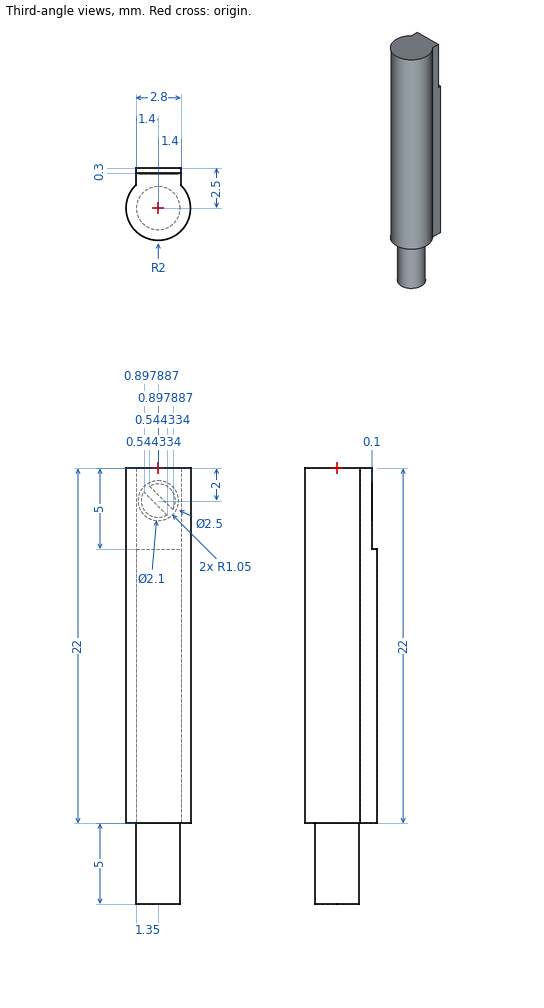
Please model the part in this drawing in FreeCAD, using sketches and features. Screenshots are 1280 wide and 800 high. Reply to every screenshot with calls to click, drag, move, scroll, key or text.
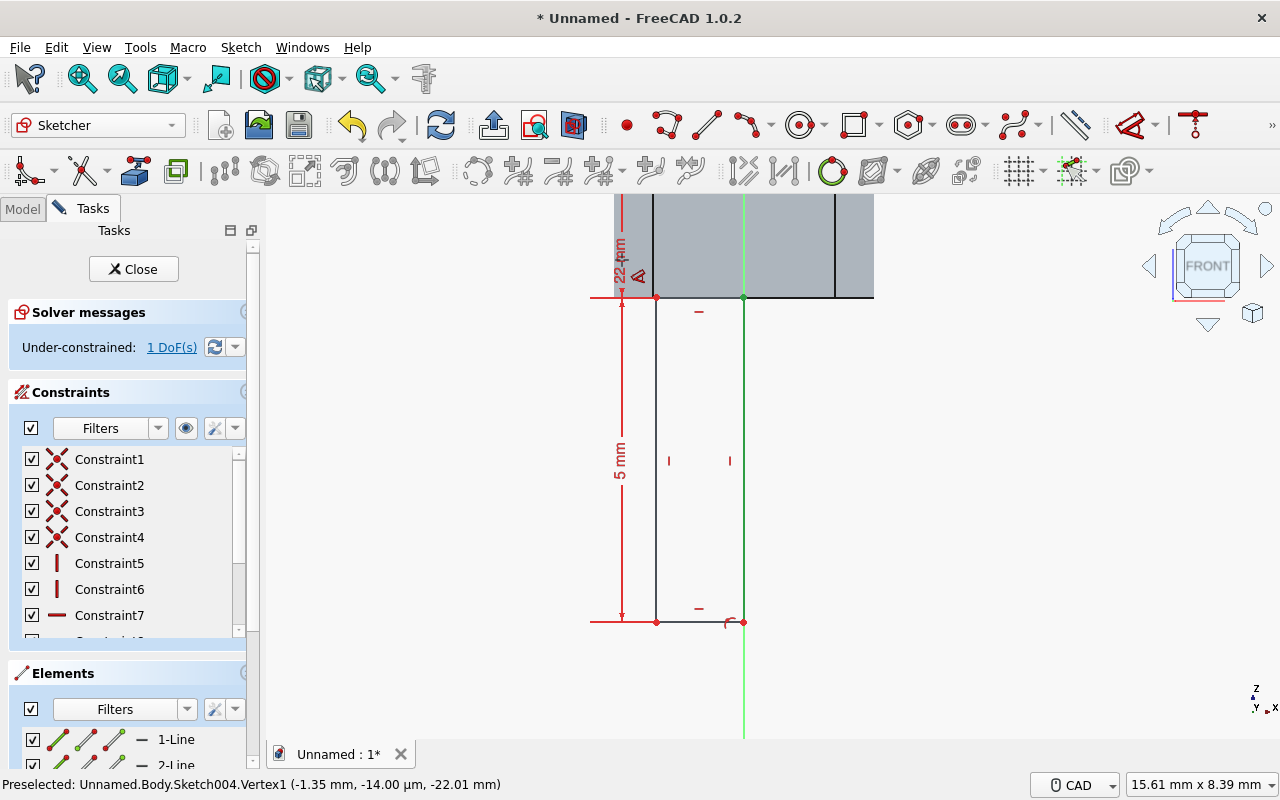
click(682, 622)
click(700, 656)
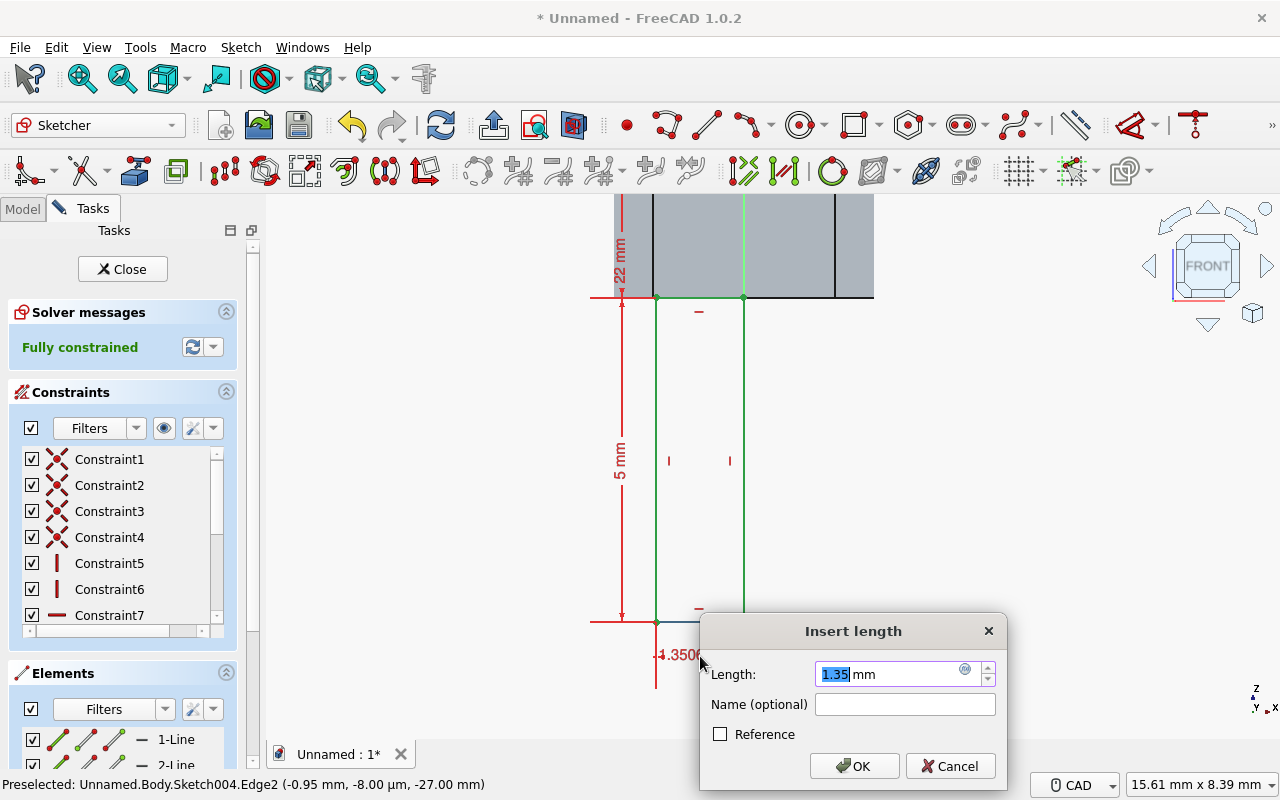
text(1.35)
key(Return)
key(Escape)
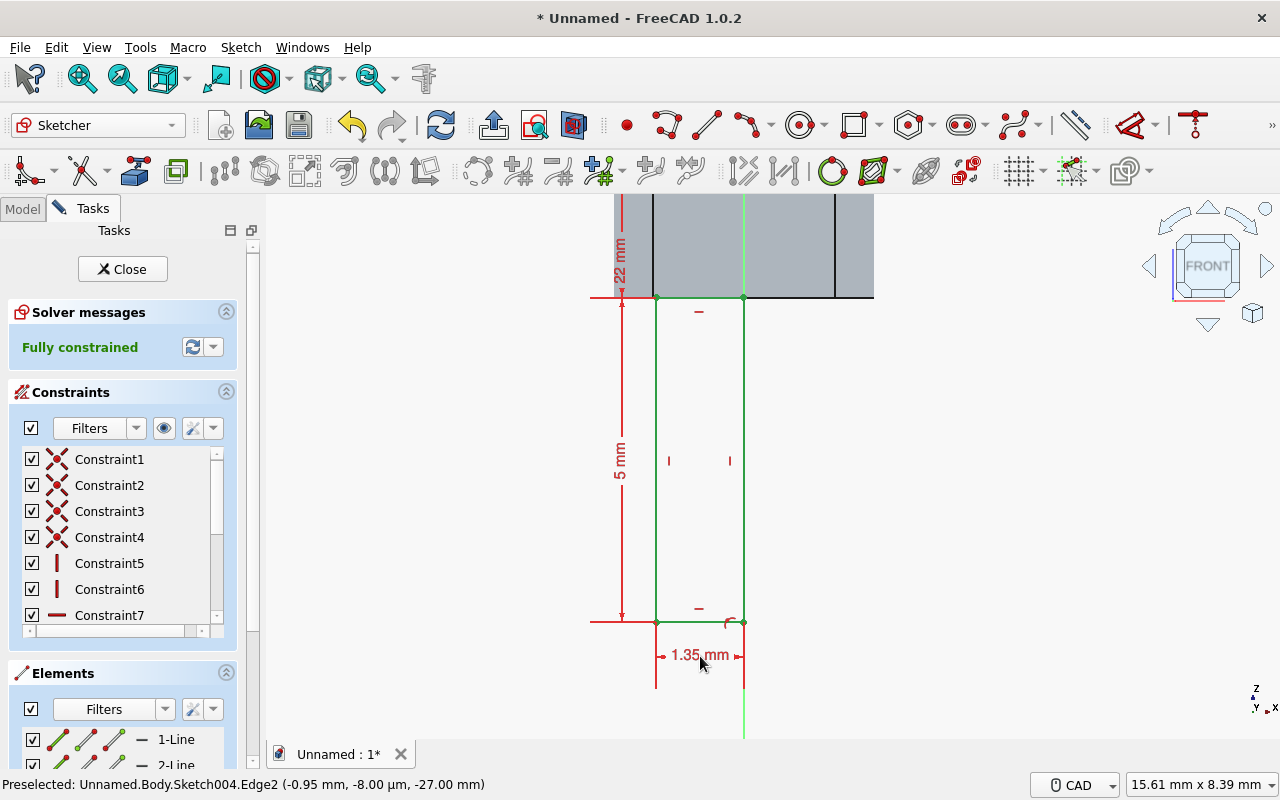
click(123, 269)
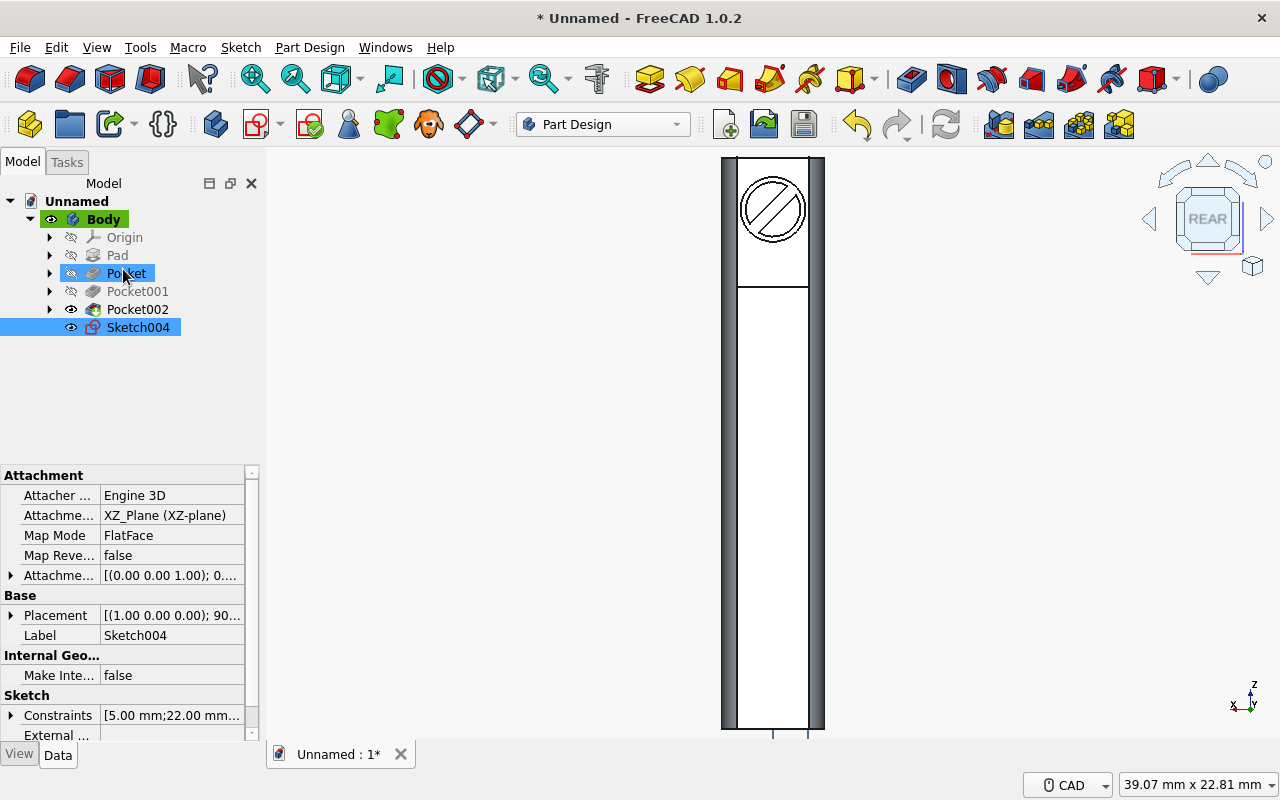
click(690, 80)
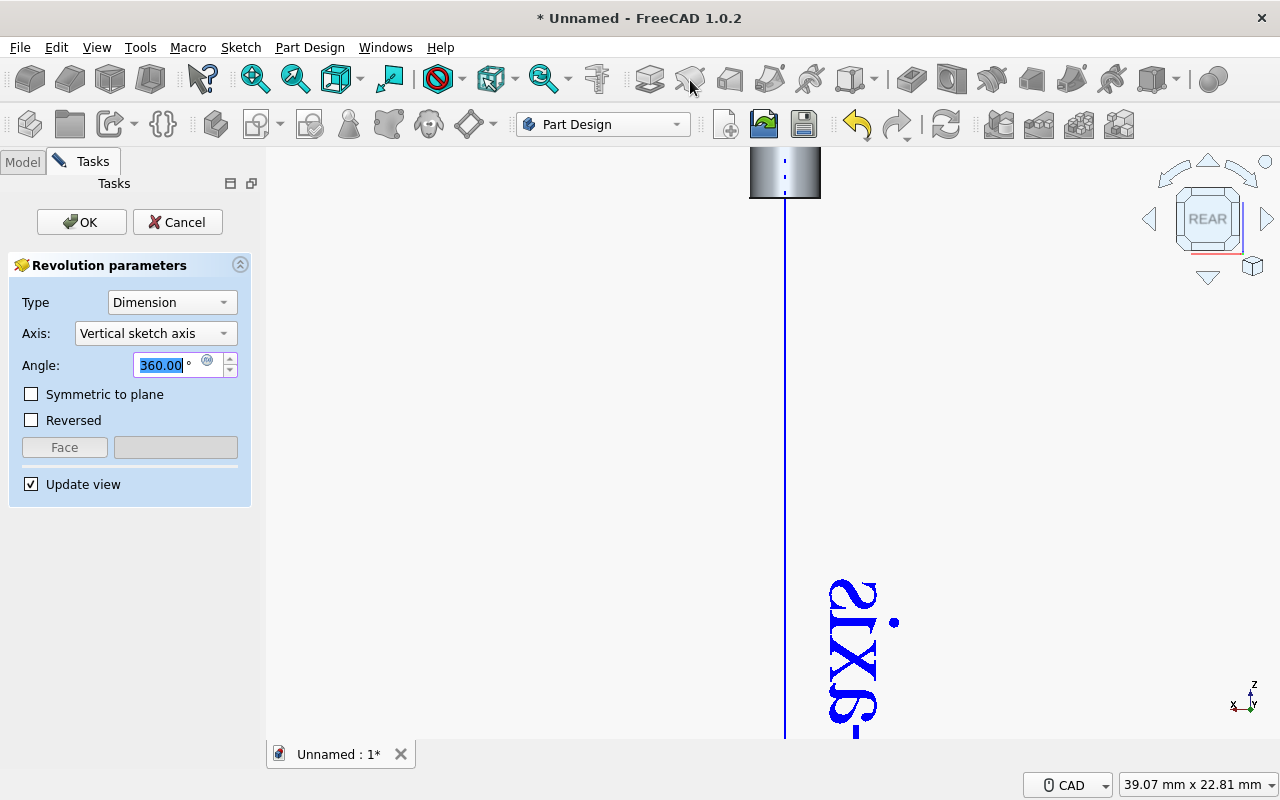
click(82, 222)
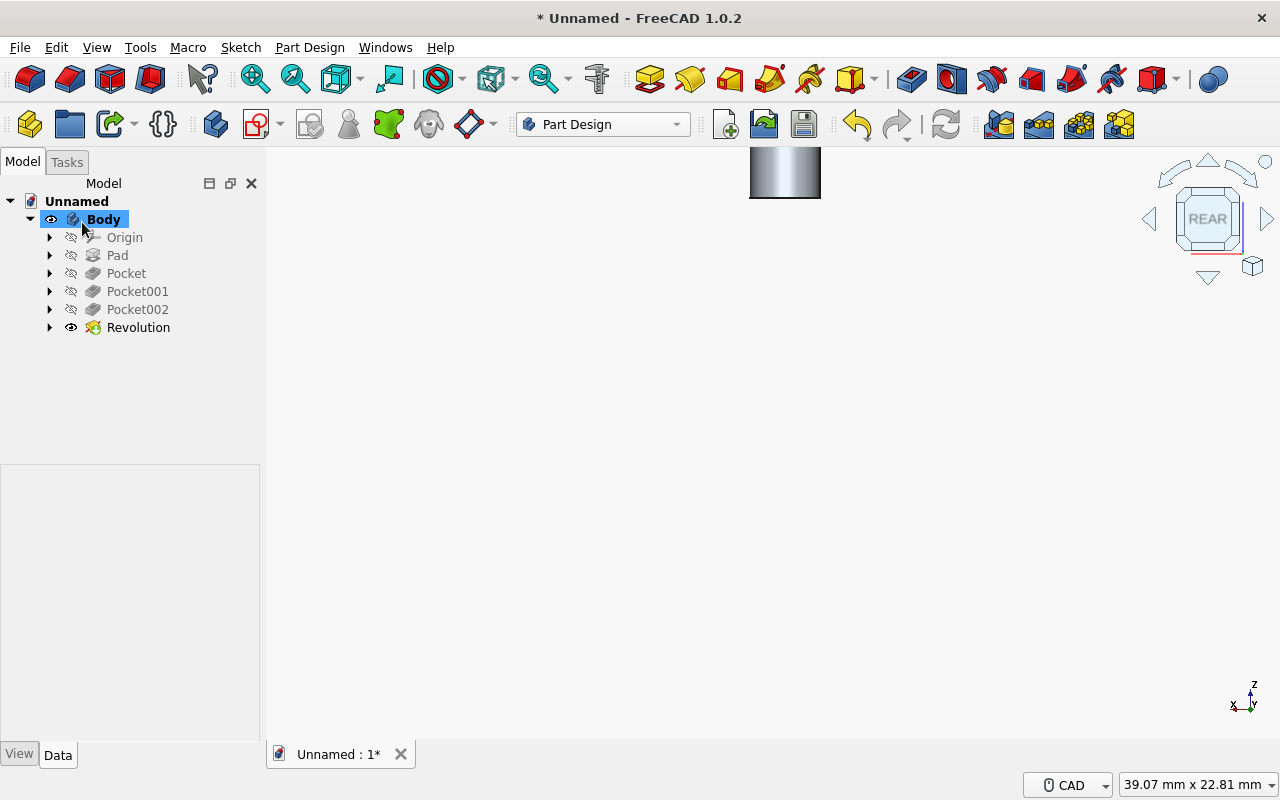
key(0)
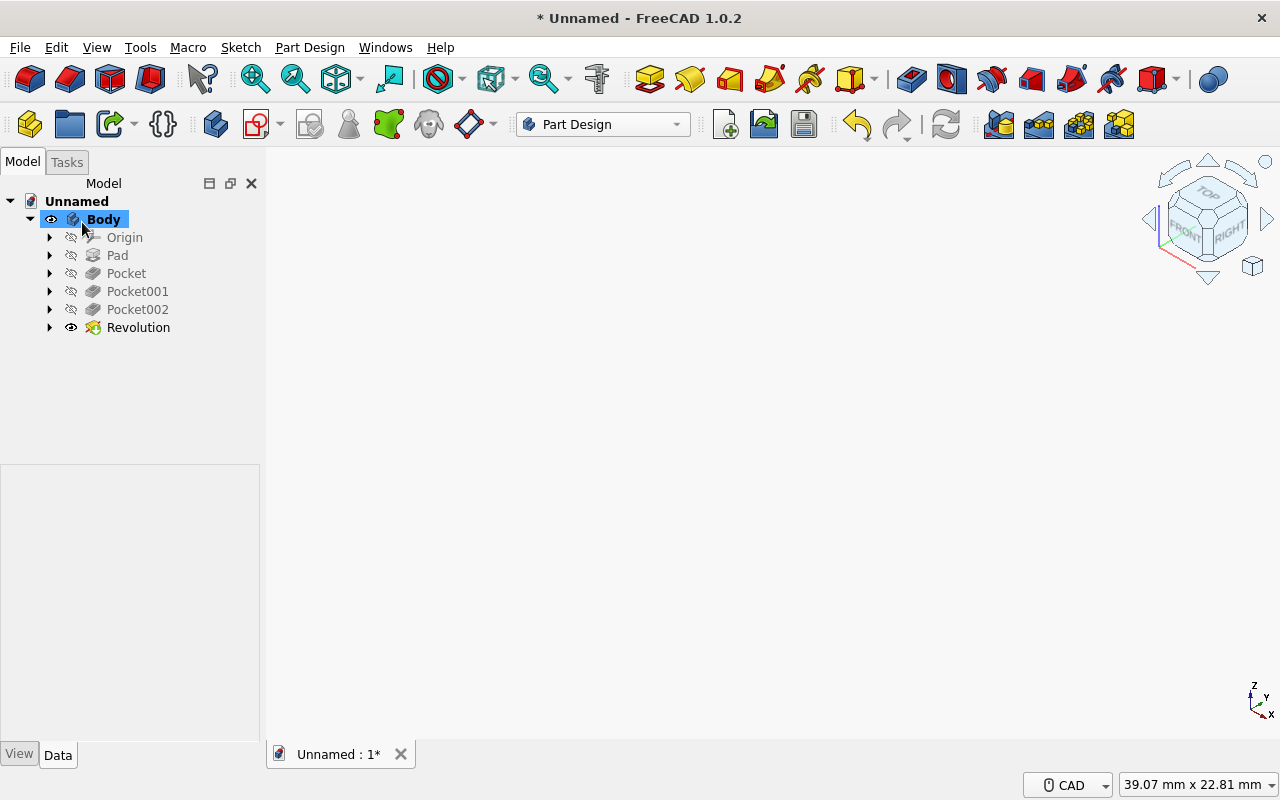
click(256, 80)